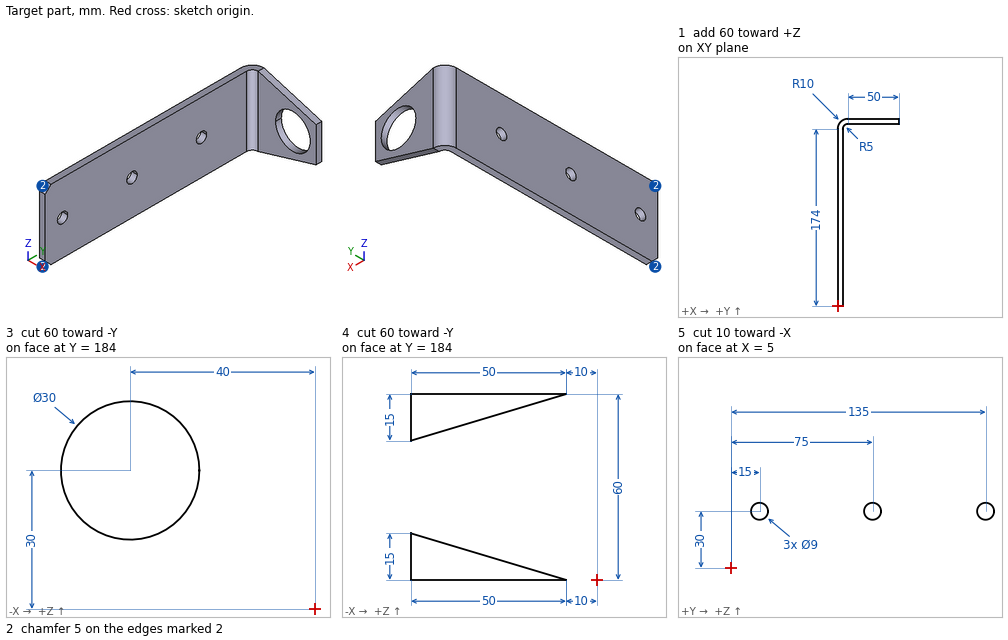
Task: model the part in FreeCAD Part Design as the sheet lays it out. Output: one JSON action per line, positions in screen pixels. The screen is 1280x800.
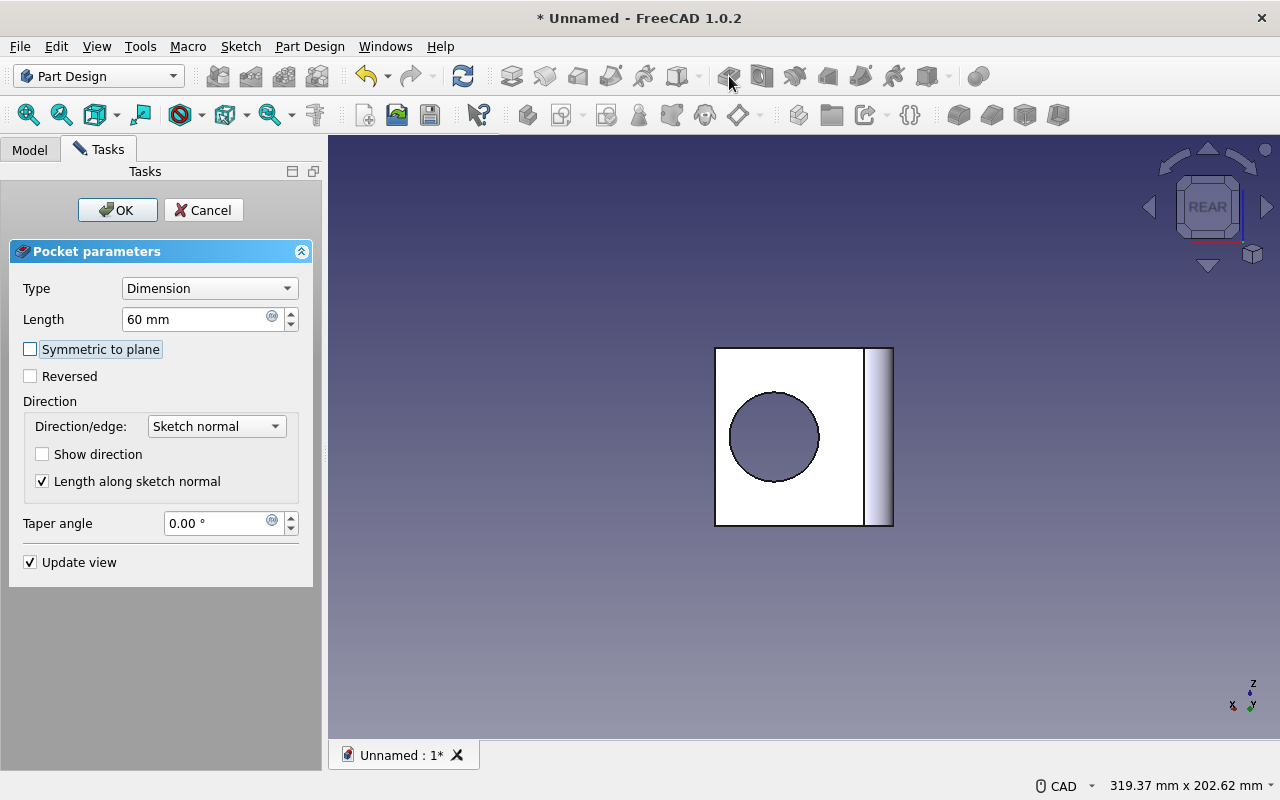
{"action": "left_click", "coordinate": [118, 210]}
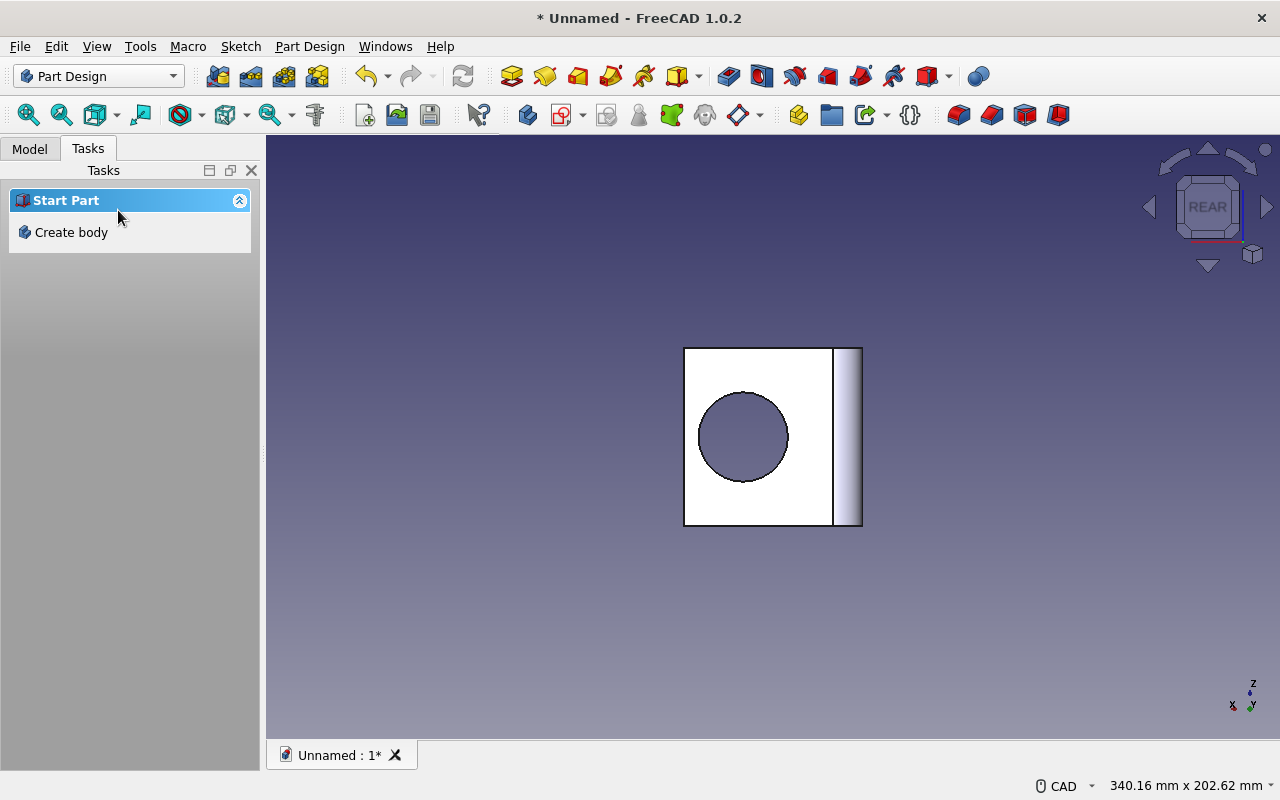
{"action": "key", "text": "v f"}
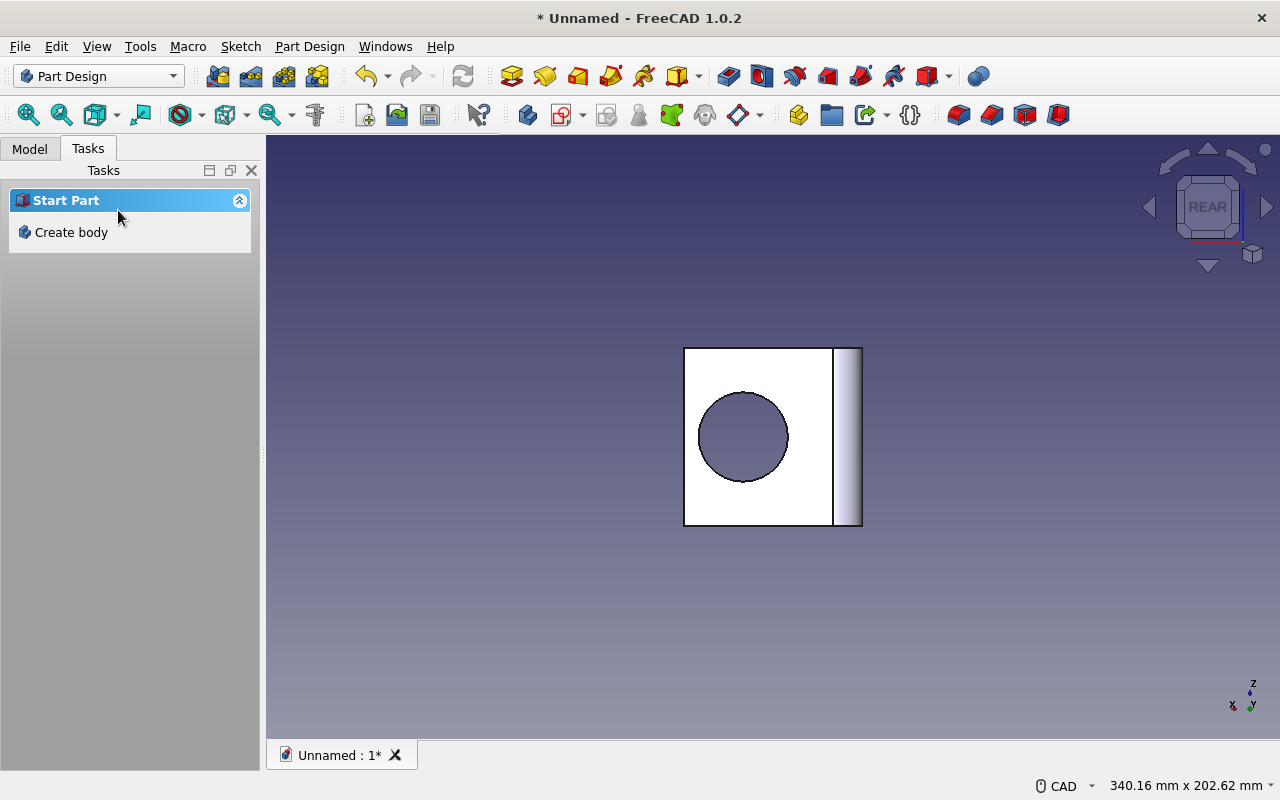
{"action": "left_click", "coordinate": [801, 385]}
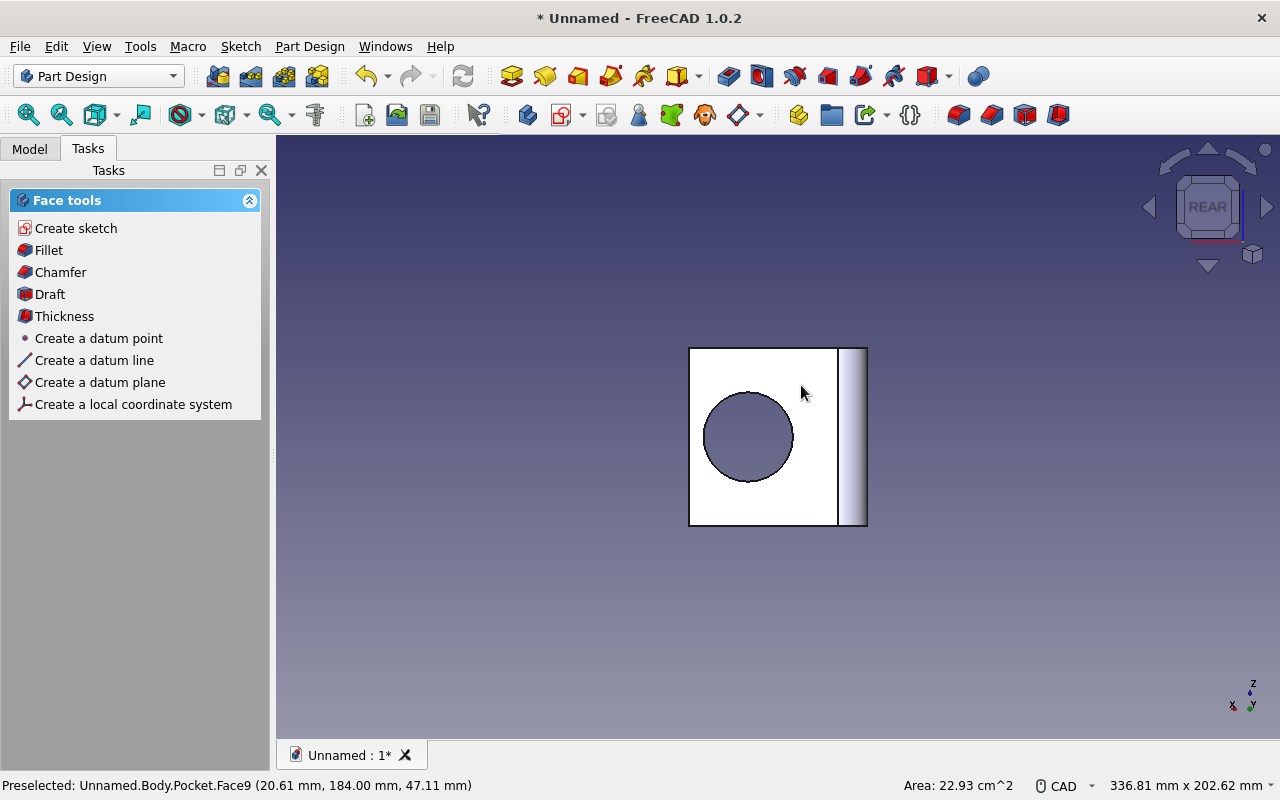
{"action": "left_click", "coordinate": [560, 116]}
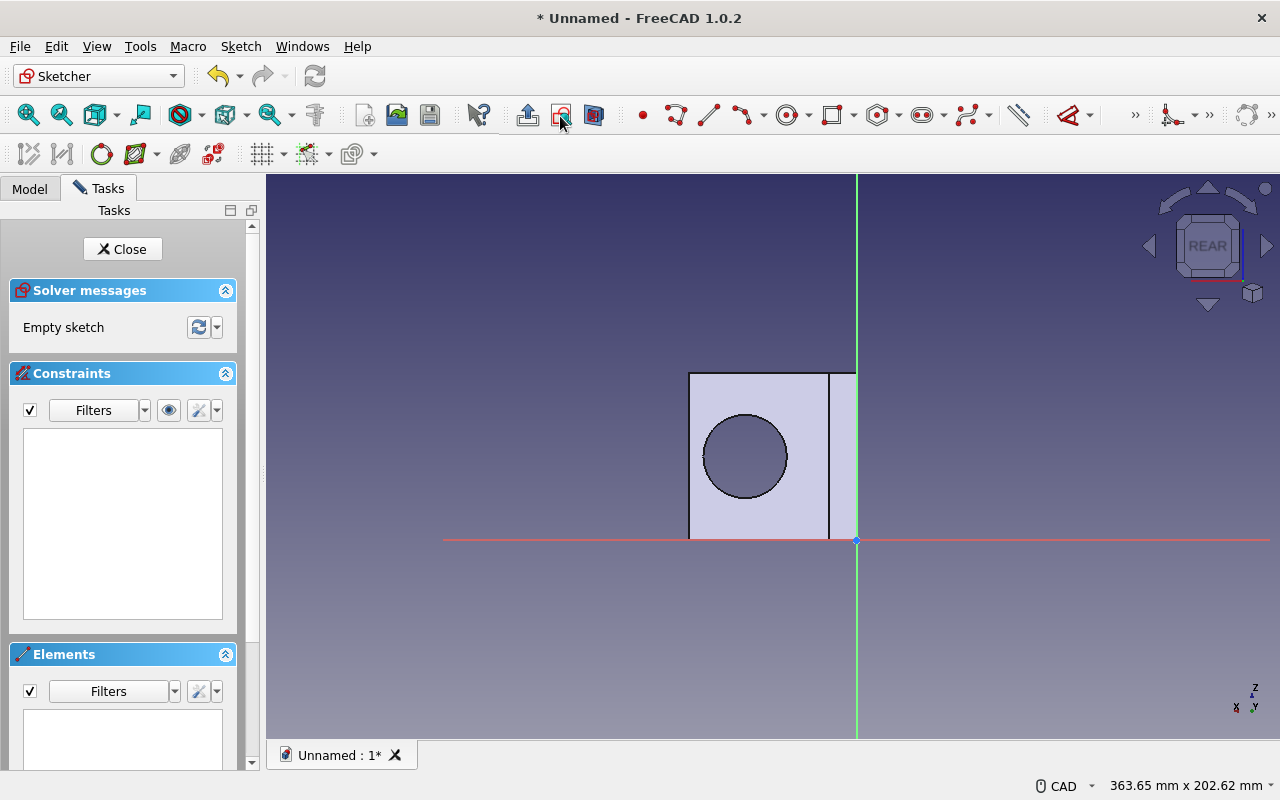
{"action": "scroll", "coordinate": [829, 457], "scroll_direction": "up", "scroll_amount": 4}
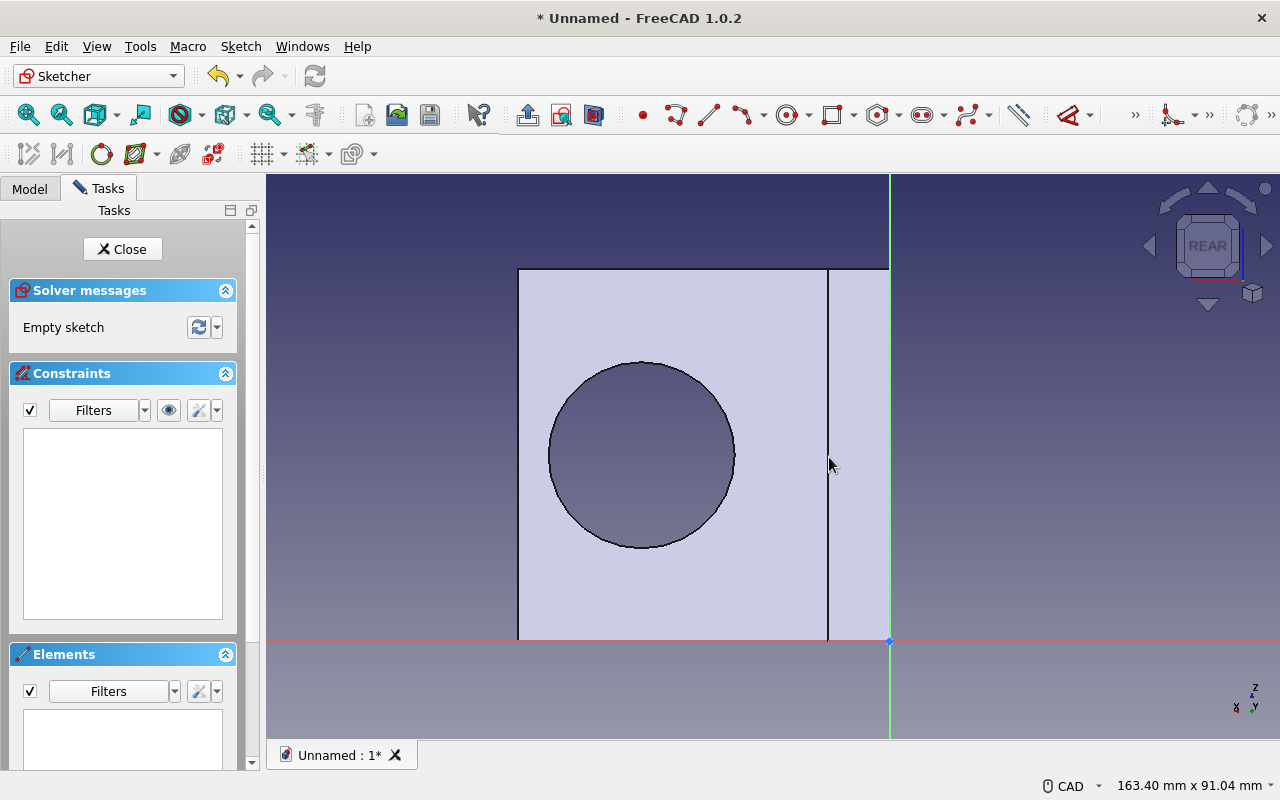
{"action": "left_click", "coordinate": [676, 116]}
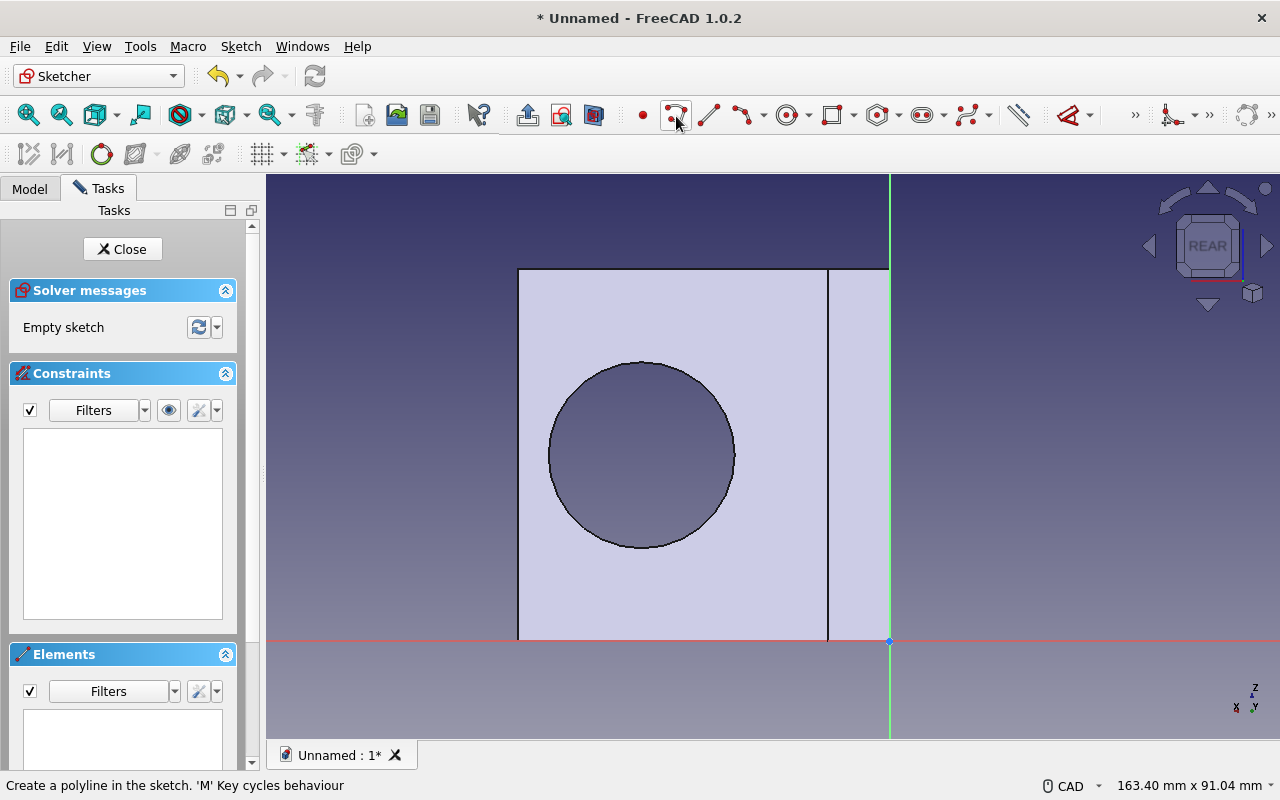
{"action": "left_click", "coordinate": [828, 641]}
{"action": "left_click", "coordinate": [518, 548]}
{"action": "left_click", "coordinate": [518, 632]}
{"action": "left_click", "coordinate": [828, 641]}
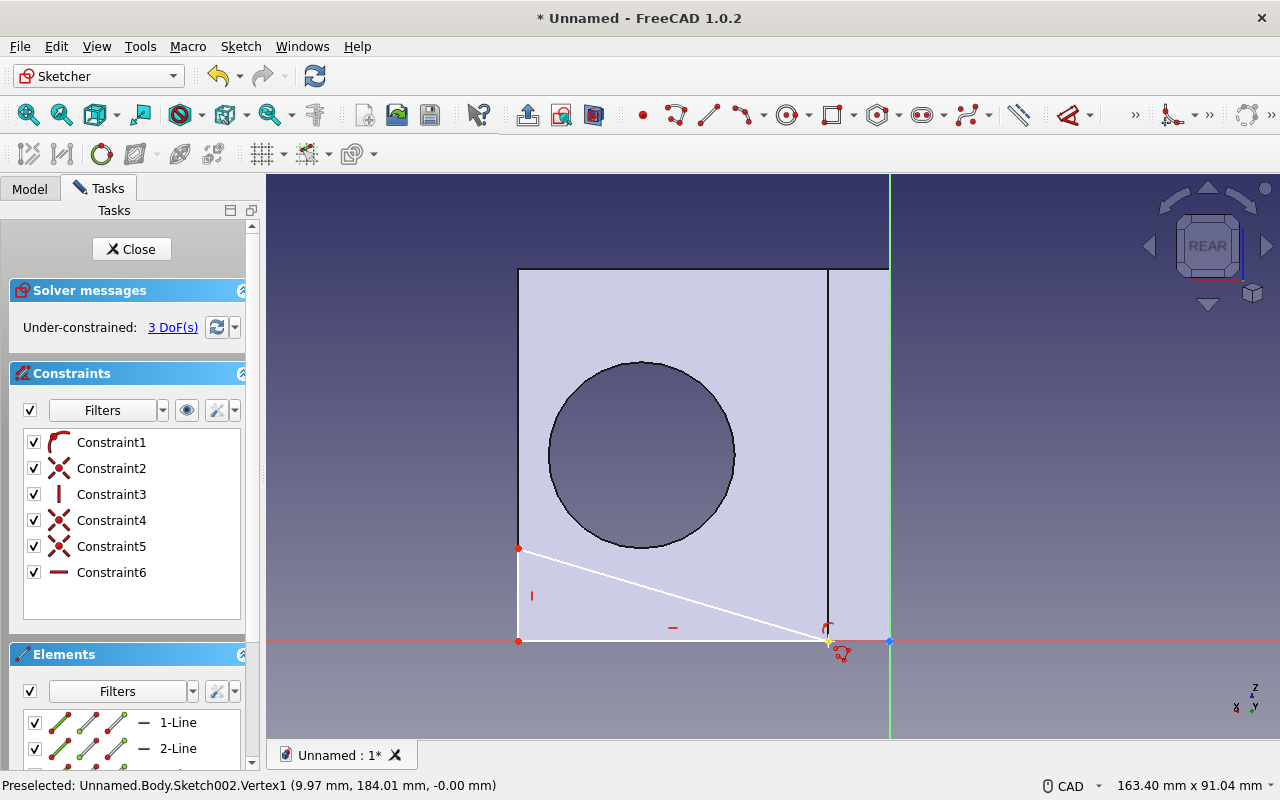
{"action": "left_click", "coordinate": [828, 269]}
{"action": "left_click", "coordinate": [518, 269]}
{"action": "left_click", "coordinate": [518, 362]}
{"action": "left_click", "coordinate": [828, 270]}
{"action": "key", "text": "Escape"}
{"action": "key", "text": "Escape"}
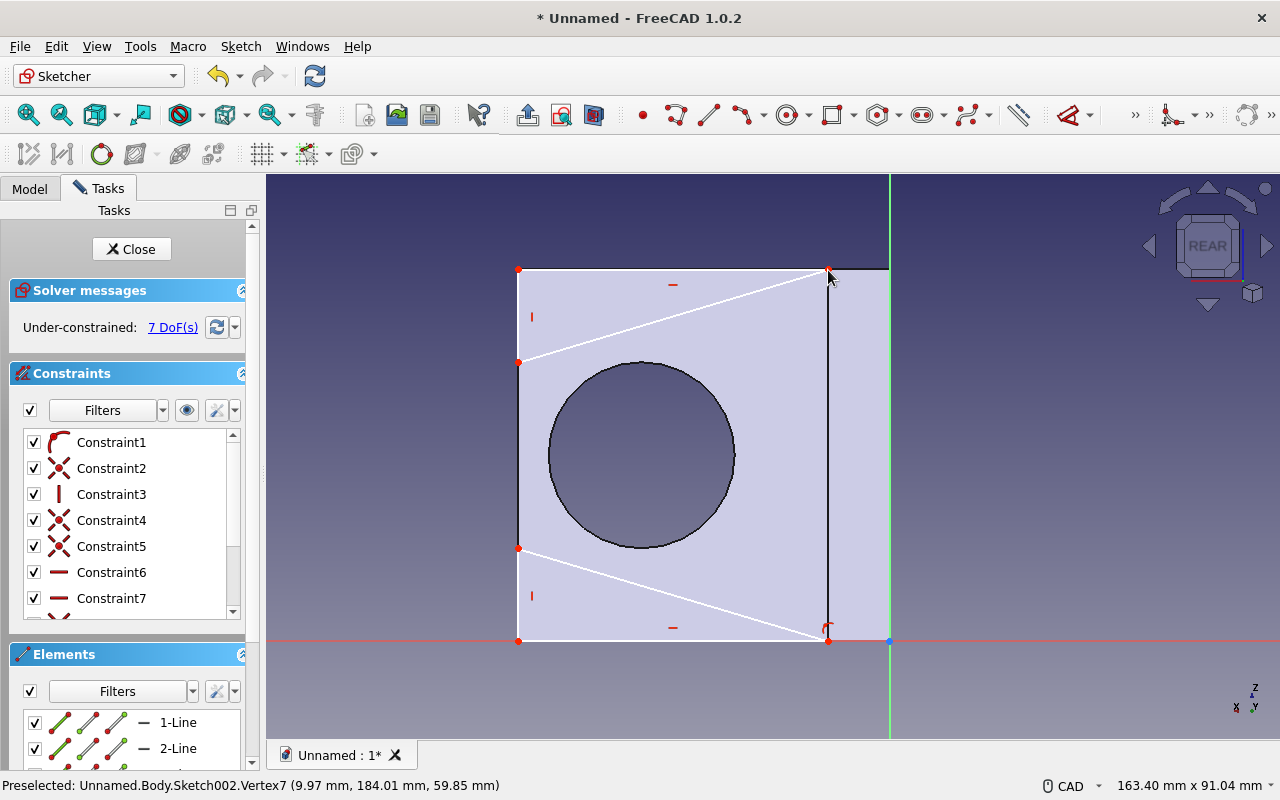
{"action": "key", "text": "d"}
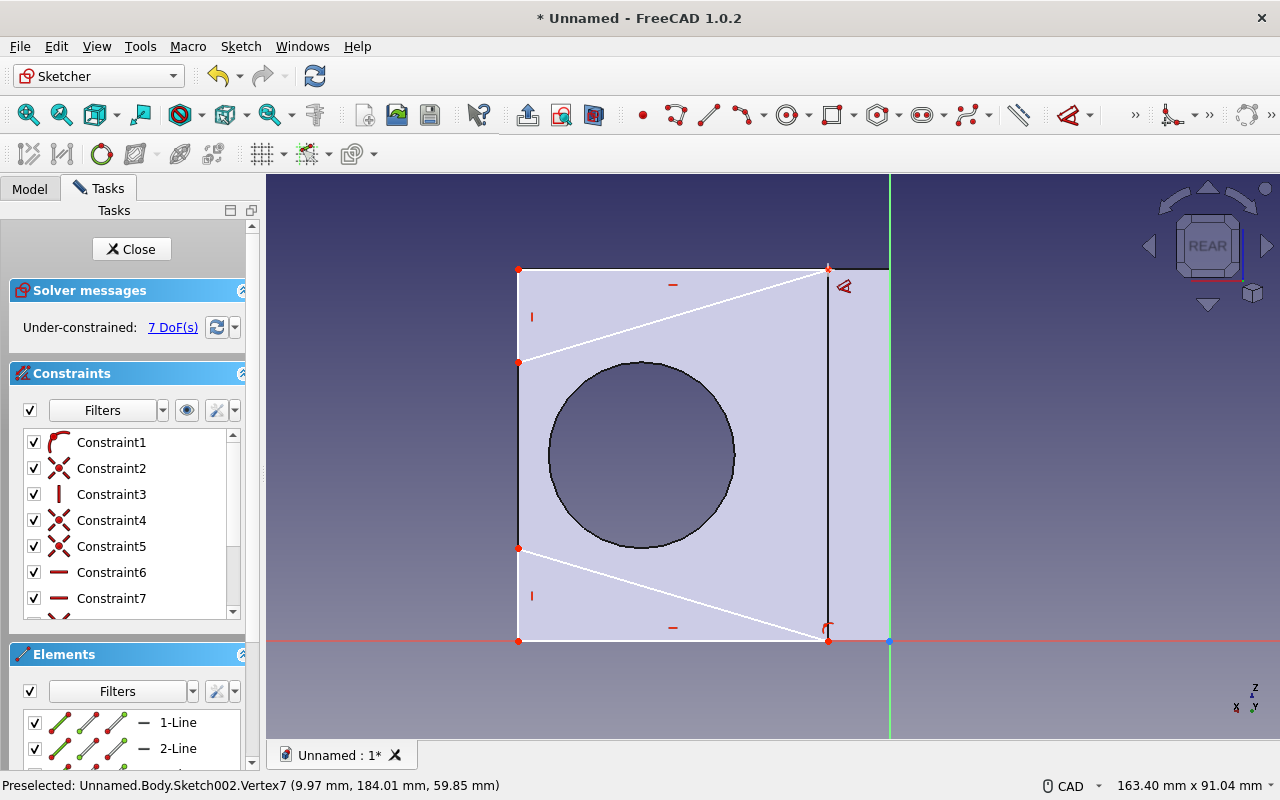
{"action": "left_click", "coordinate": [518, 577]}
{"action": "left_click", "coordinate": [484, 595]}